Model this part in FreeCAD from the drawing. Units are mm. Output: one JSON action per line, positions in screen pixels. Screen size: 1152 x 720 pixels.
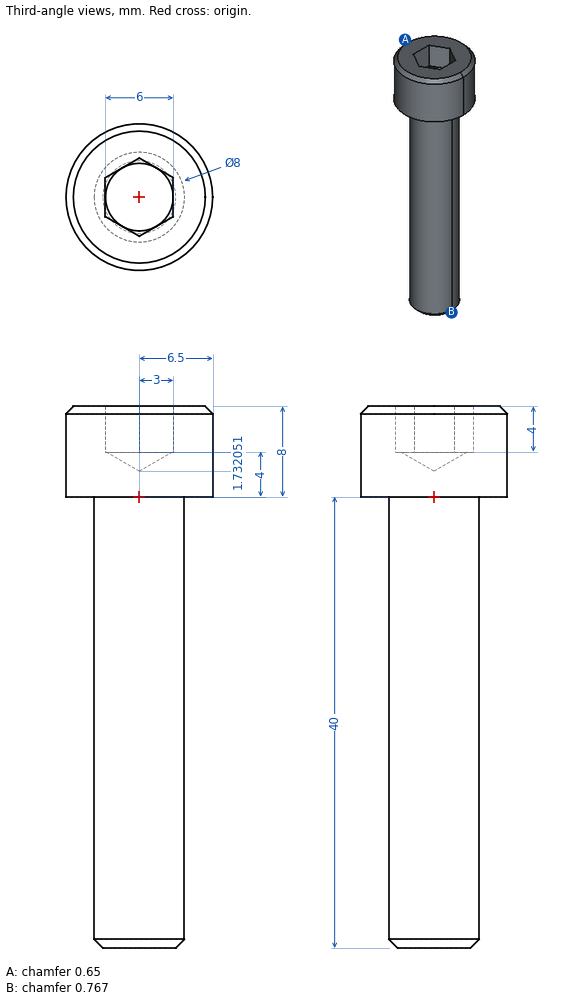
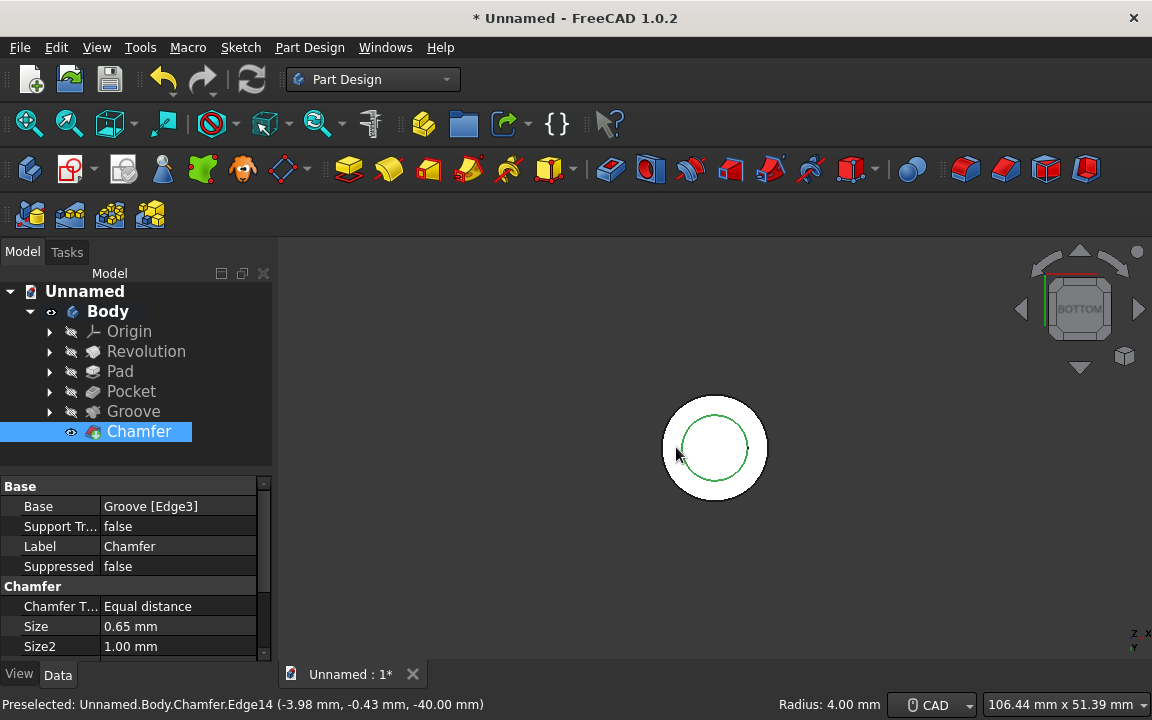
{"action": "left_click", "coordinate": [1006, 170]}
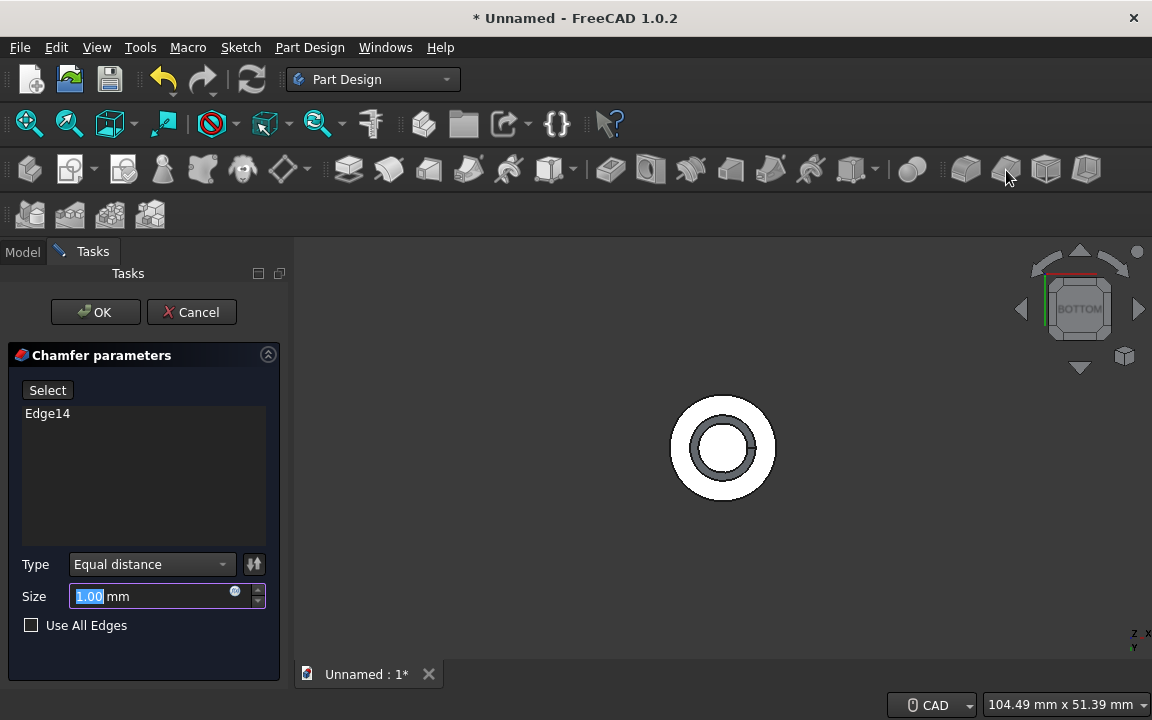
{"action": "type", "text": "0.767"}
{"action": "key", "text": "Tab"}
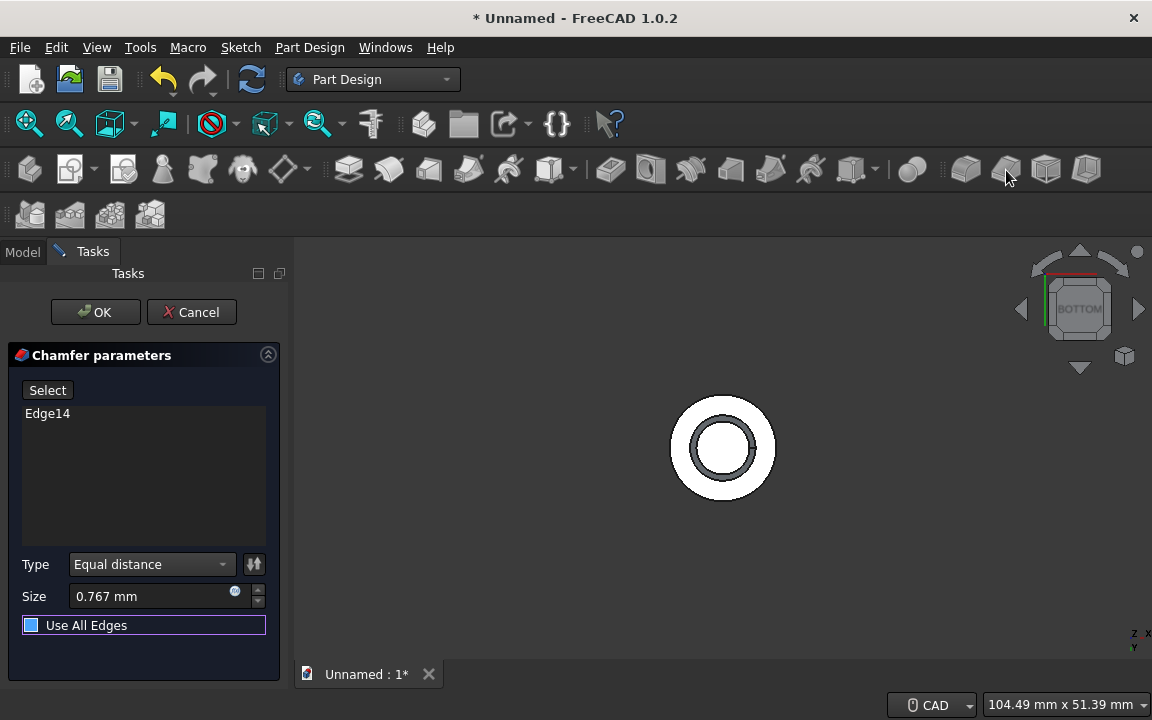
{"action": "left_click", "coordinate": [96, 312]}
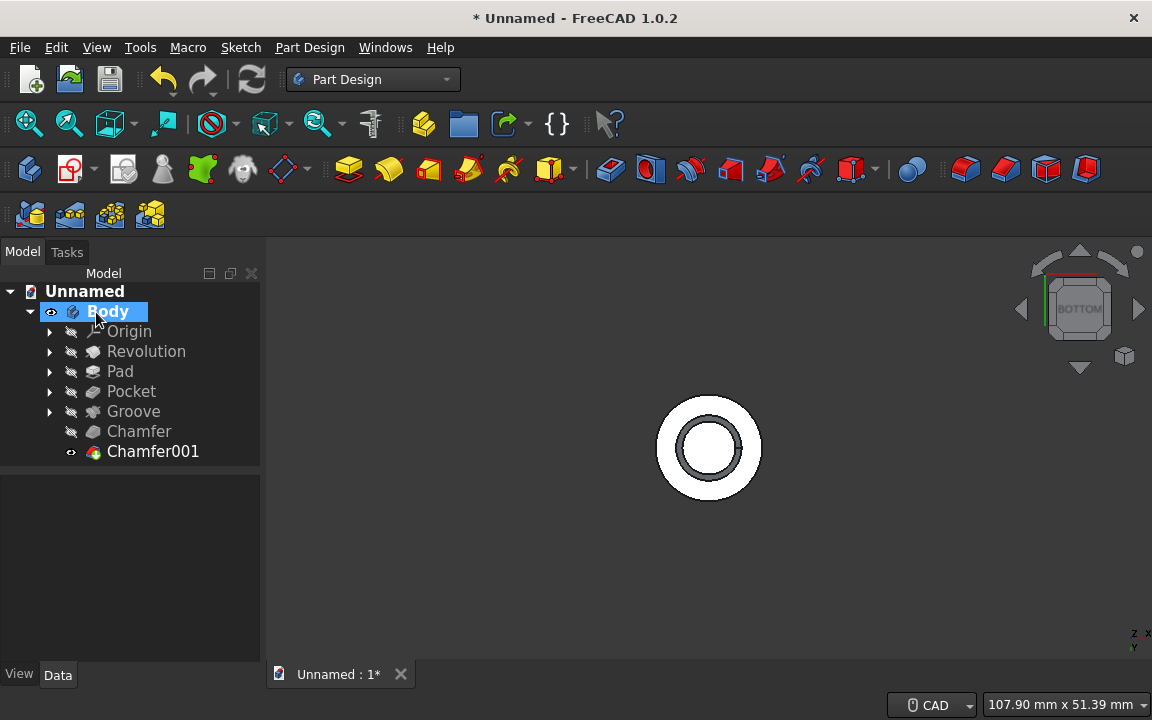
{"action": "key", "text": "0"}